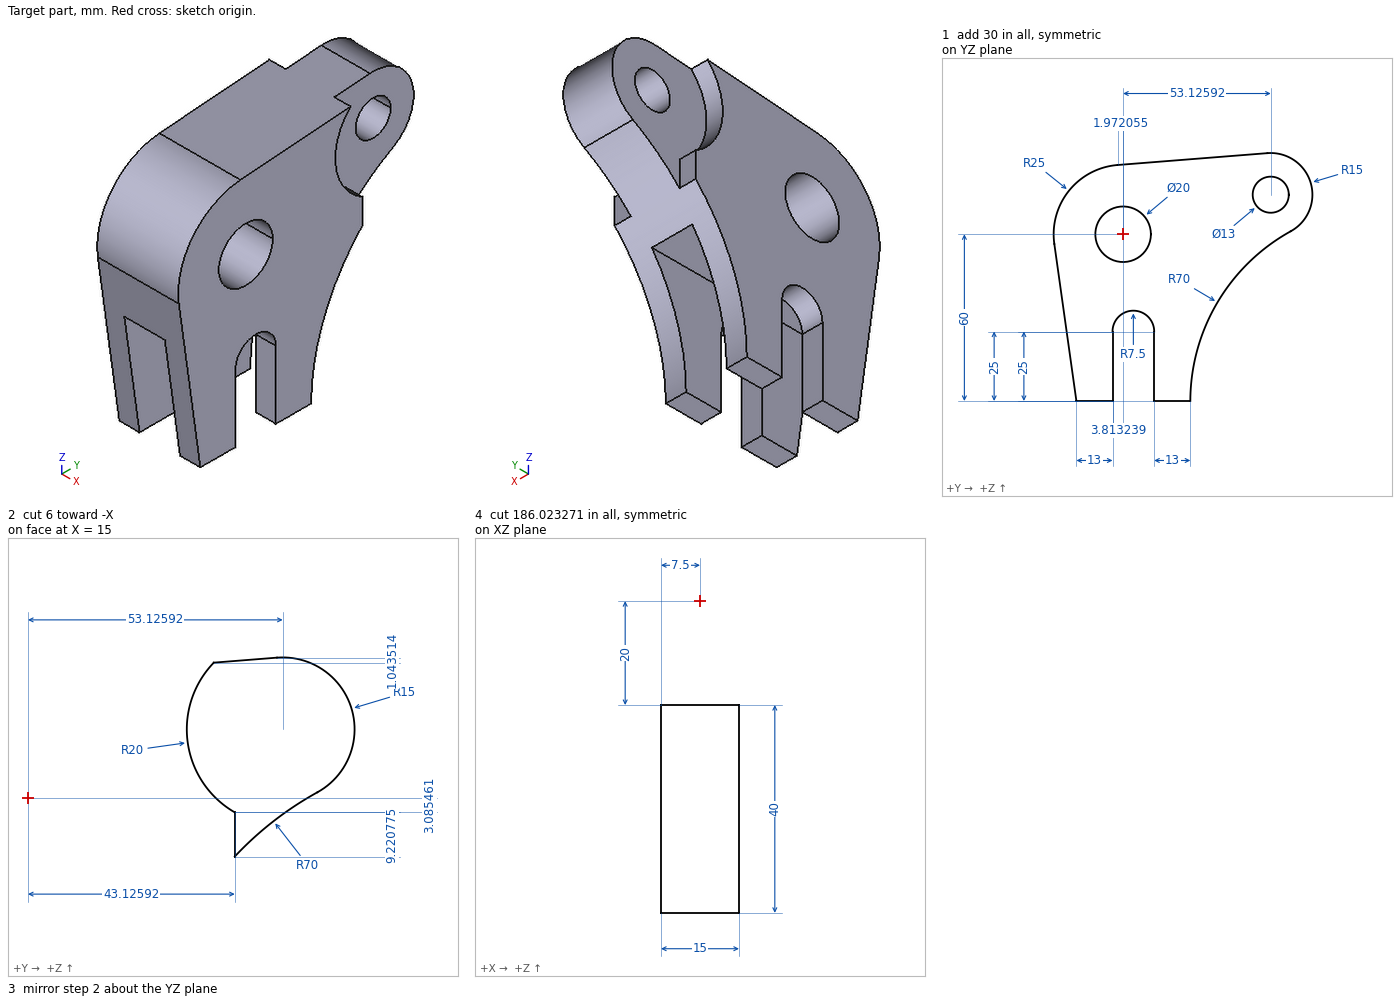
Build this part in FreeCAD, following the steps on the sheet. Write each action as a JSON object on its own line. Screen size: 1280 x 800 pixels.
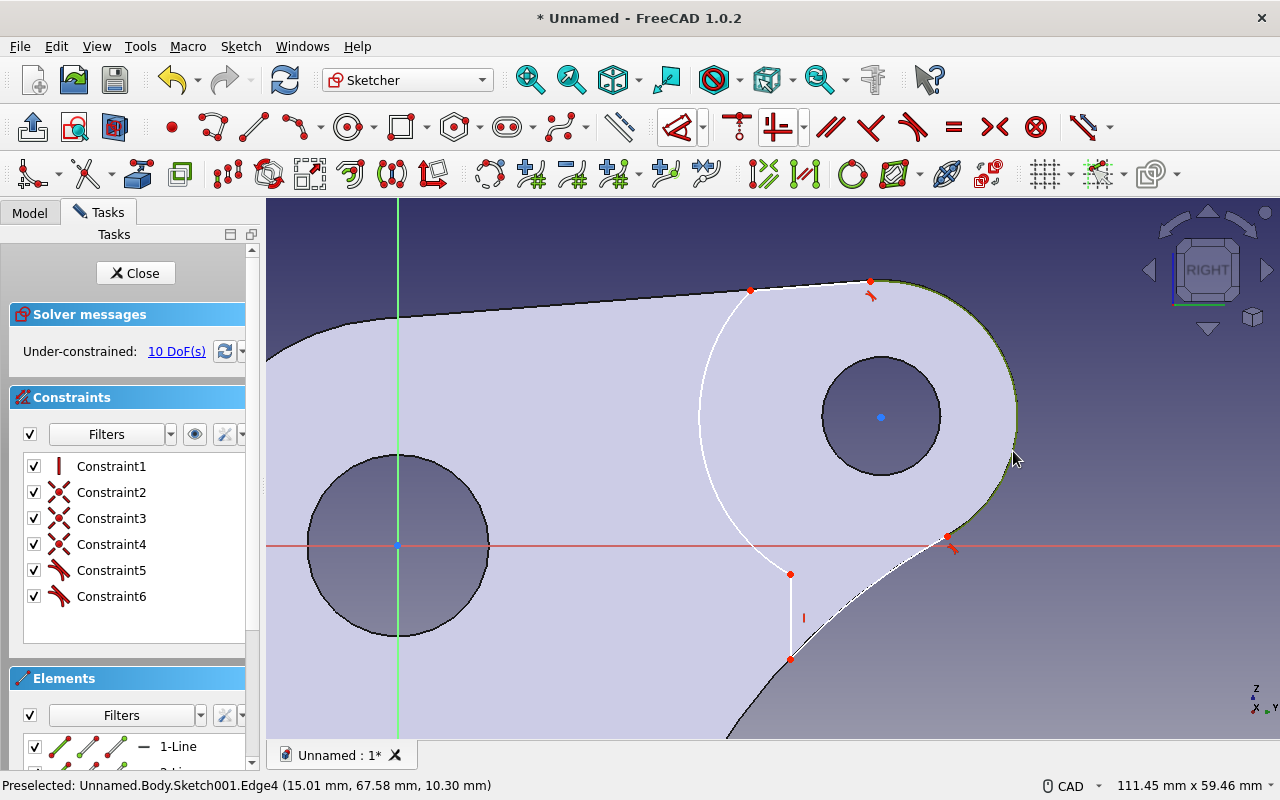
{"action": "left_click", "coordinate": [704, 377]}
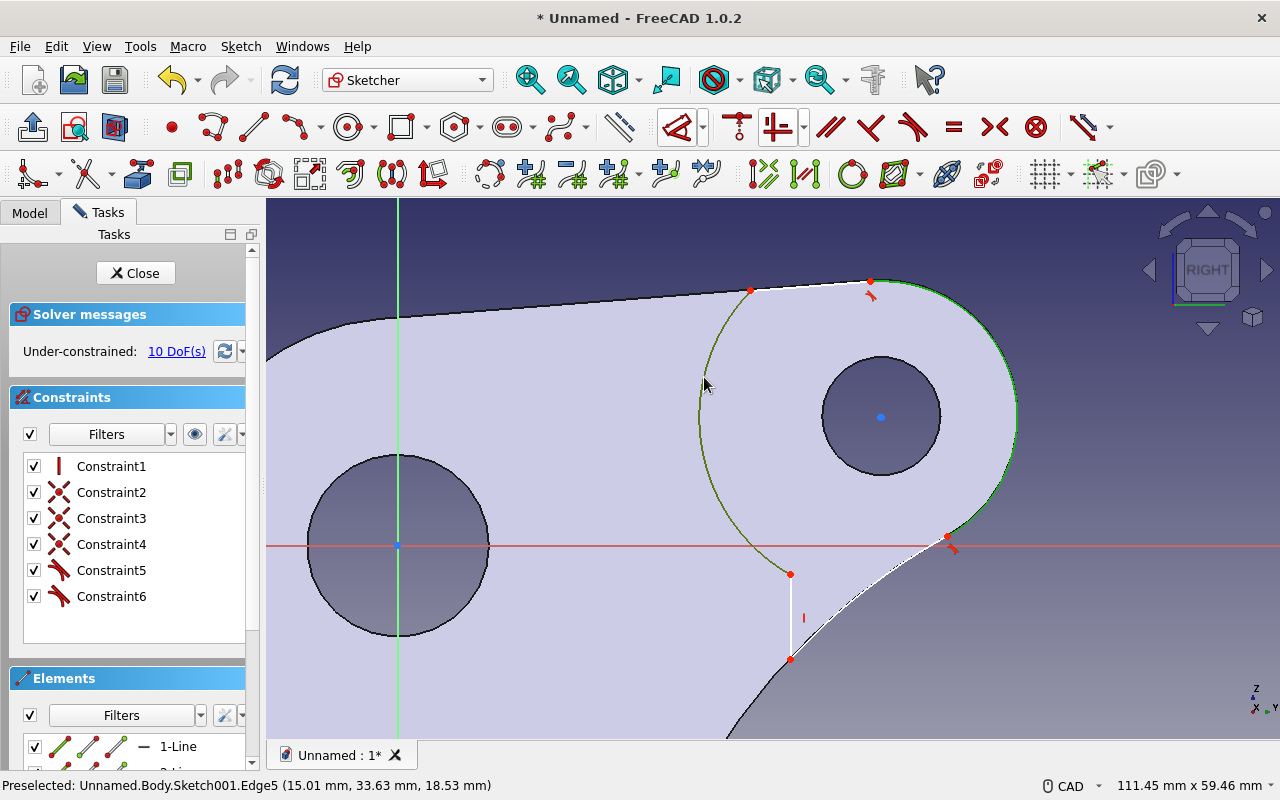
{"action": "left_click", "coordinate": [737, 128]}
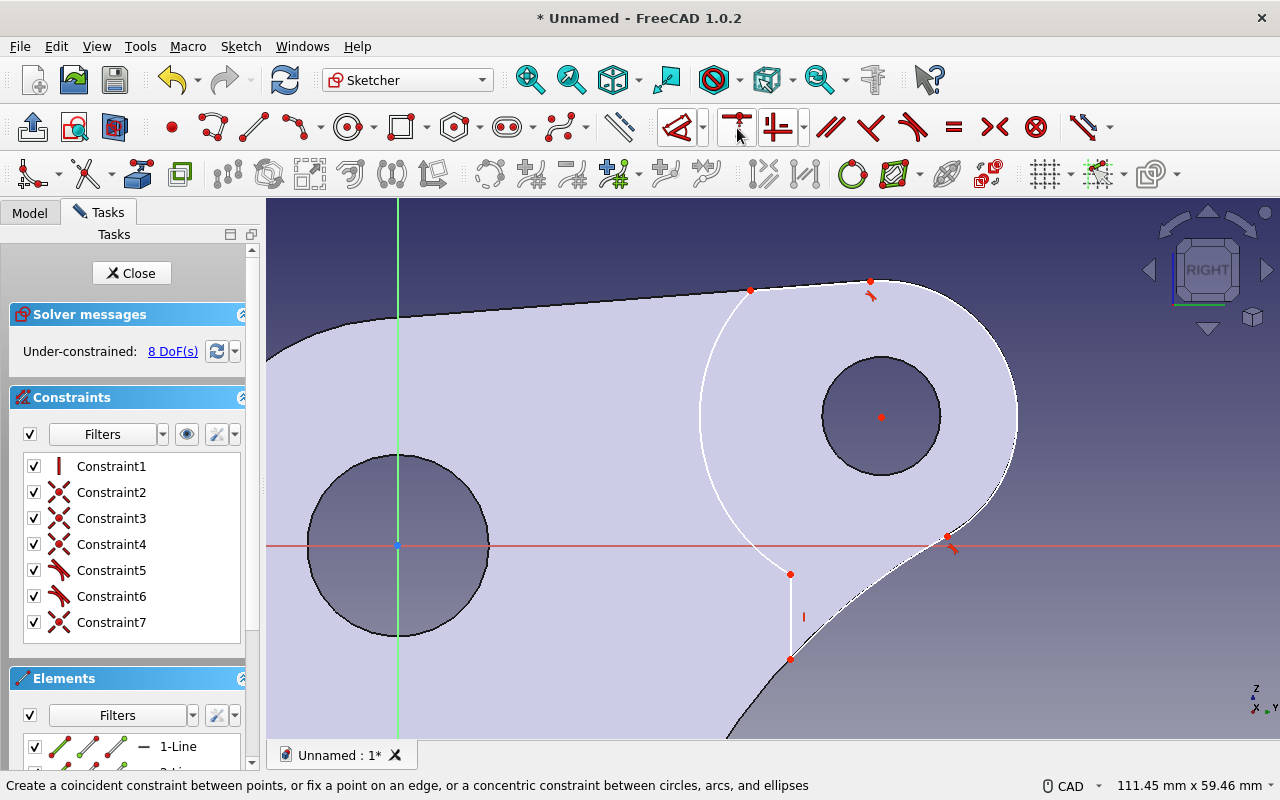
{"action": "left_click", "coordinate": [896, 568]}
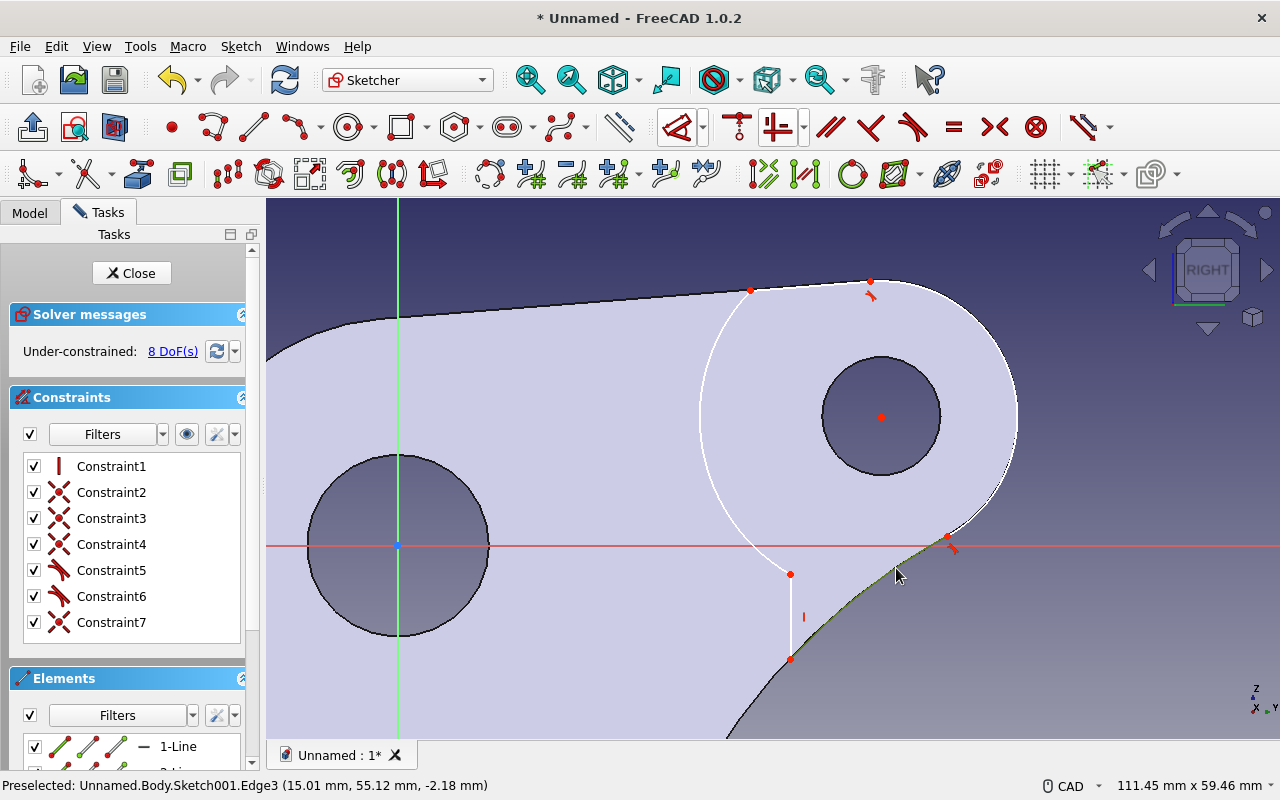
{"action": "left_click", "coordinate": [702, 128]}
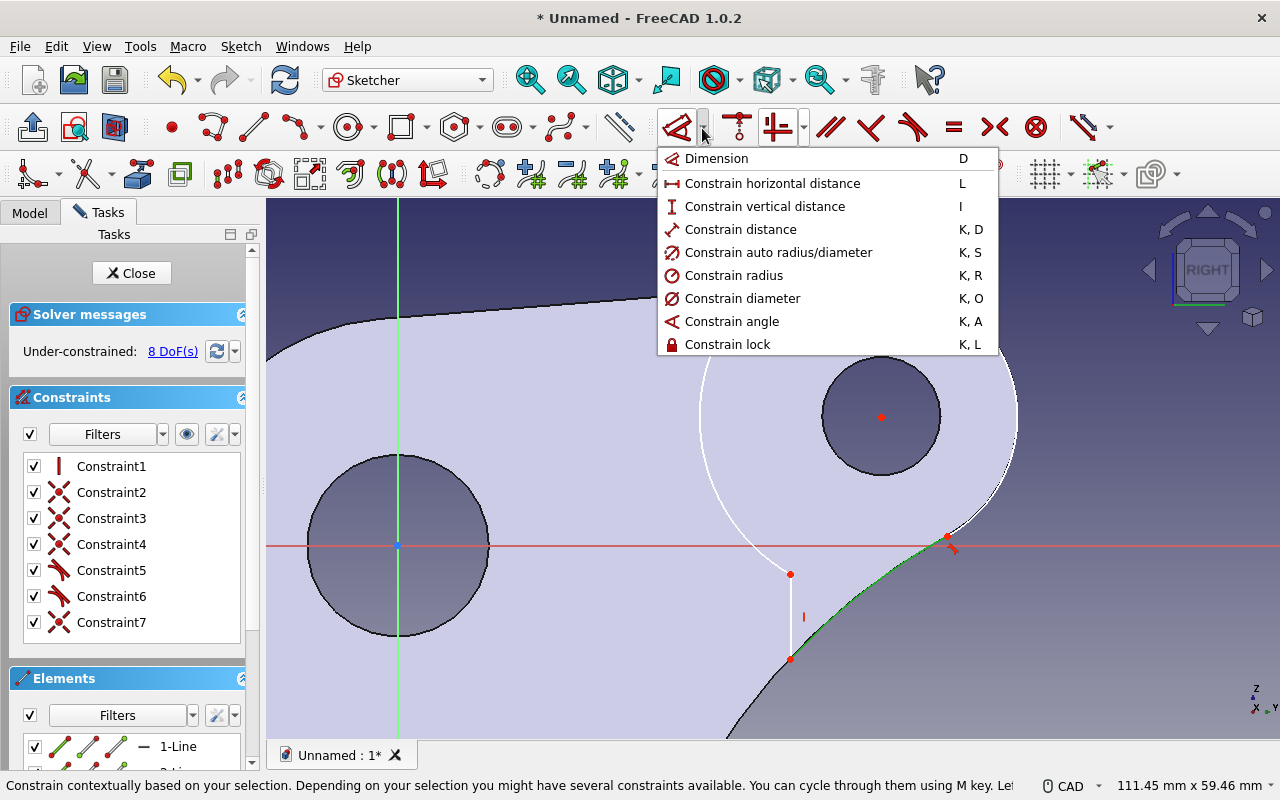
{"action": "left_click", "coordinate": [828, 276]}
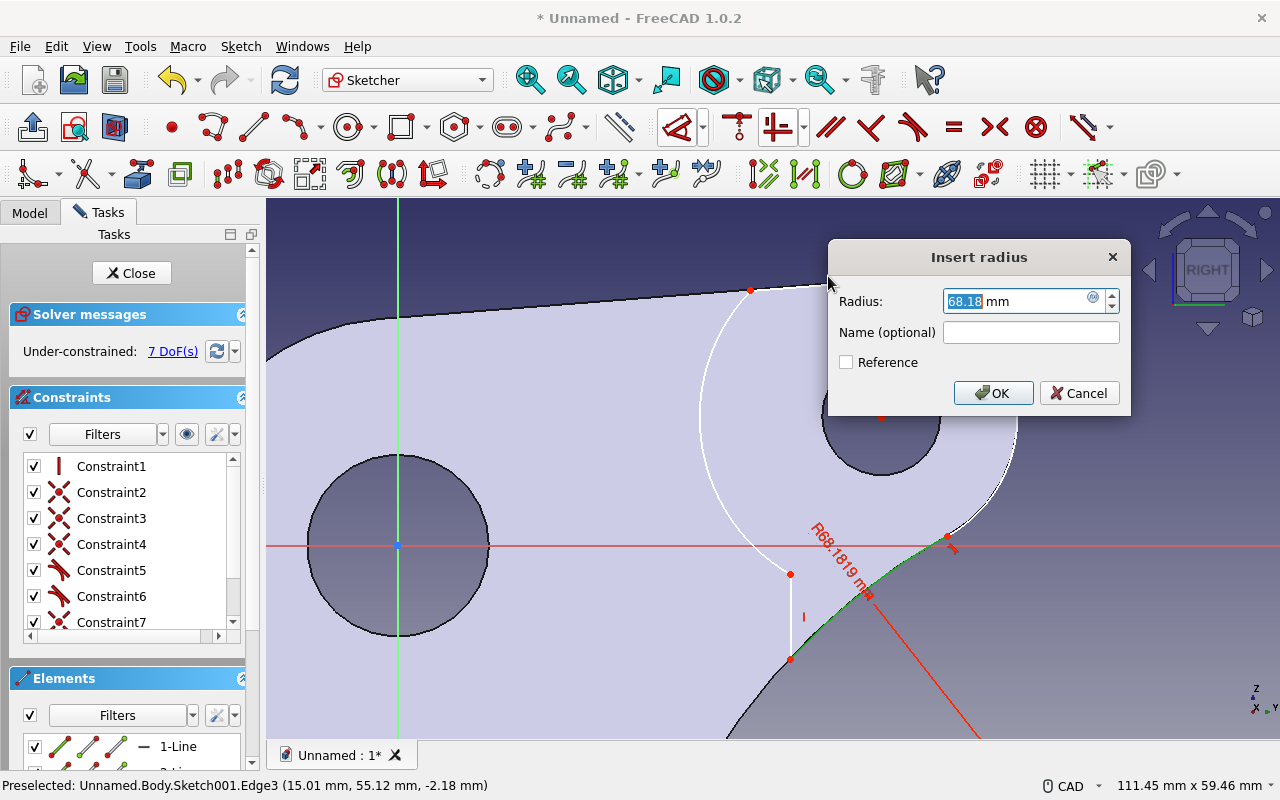
{"action": "type", "text": "70"}
{"action": "key", "text": "Return"}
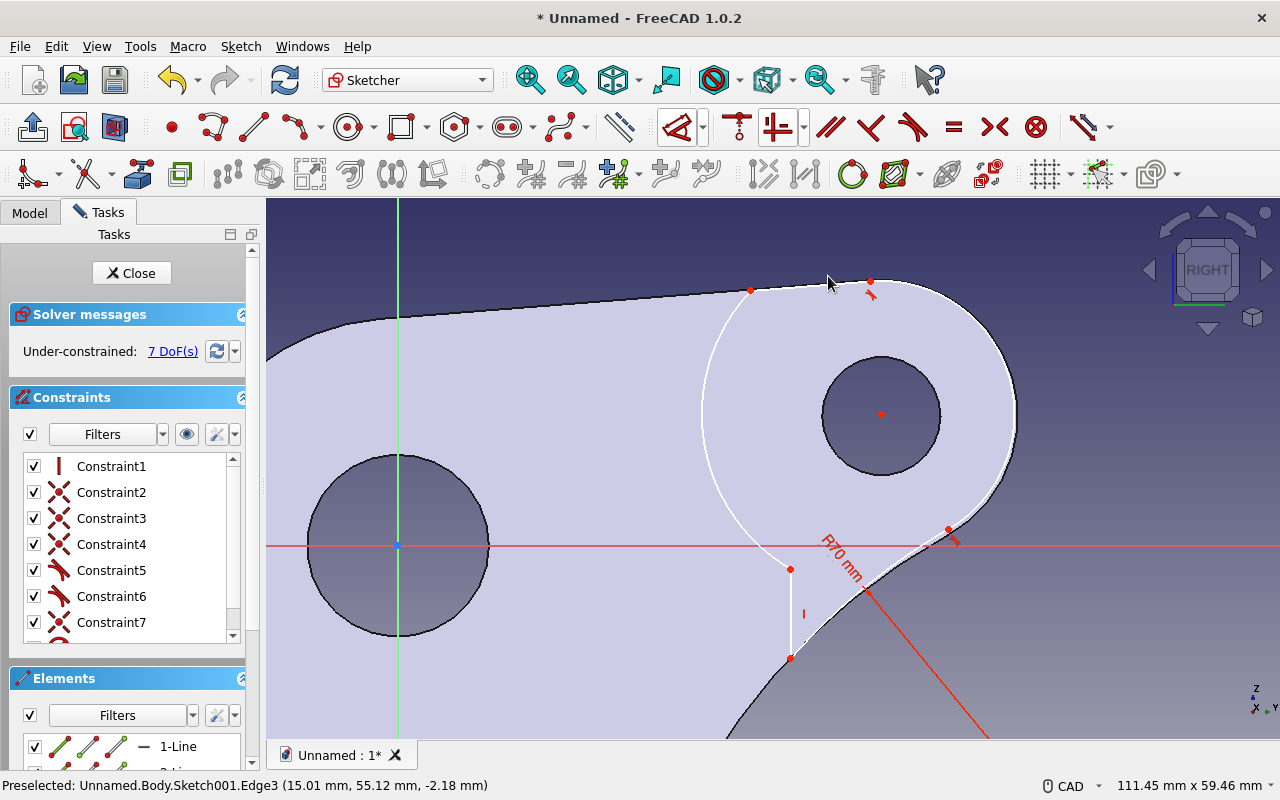
{"action": "left_click", "coordinate": [1011, 445]}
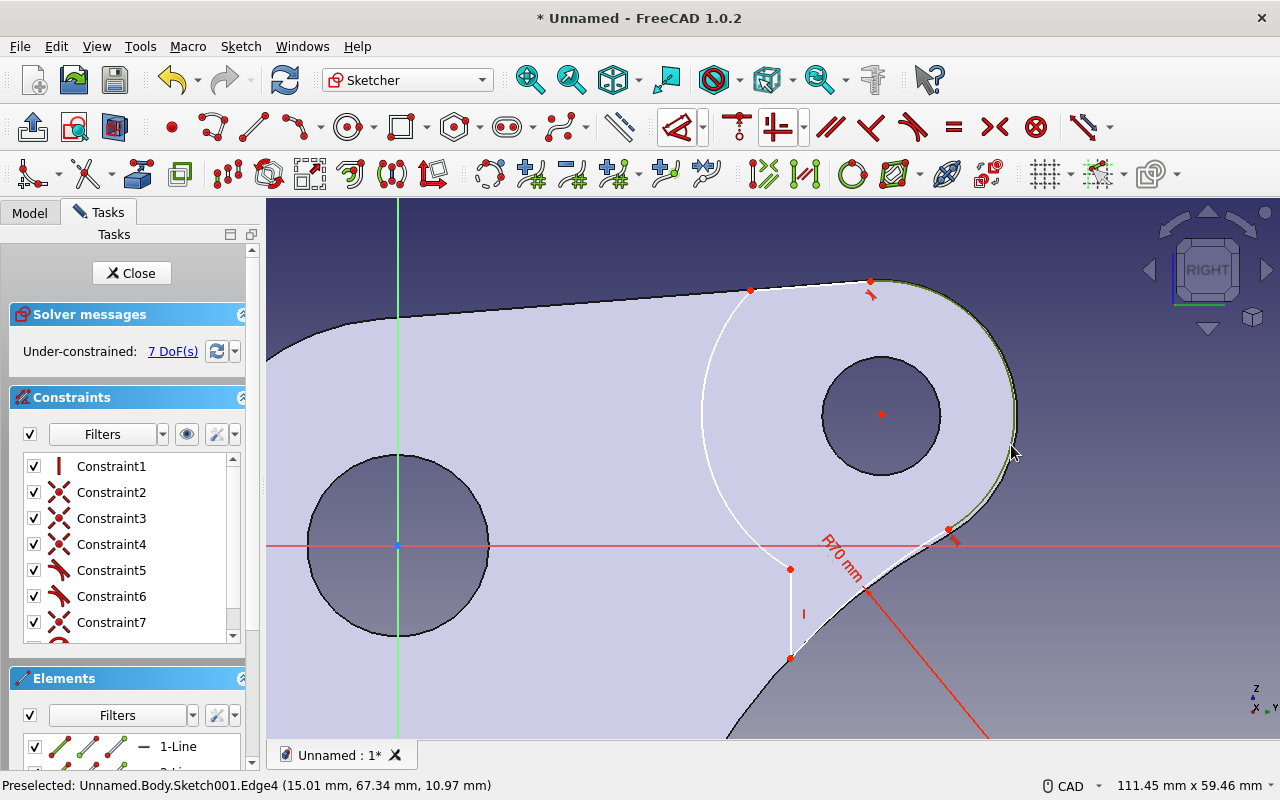
{"action": "key", "text": "k r"}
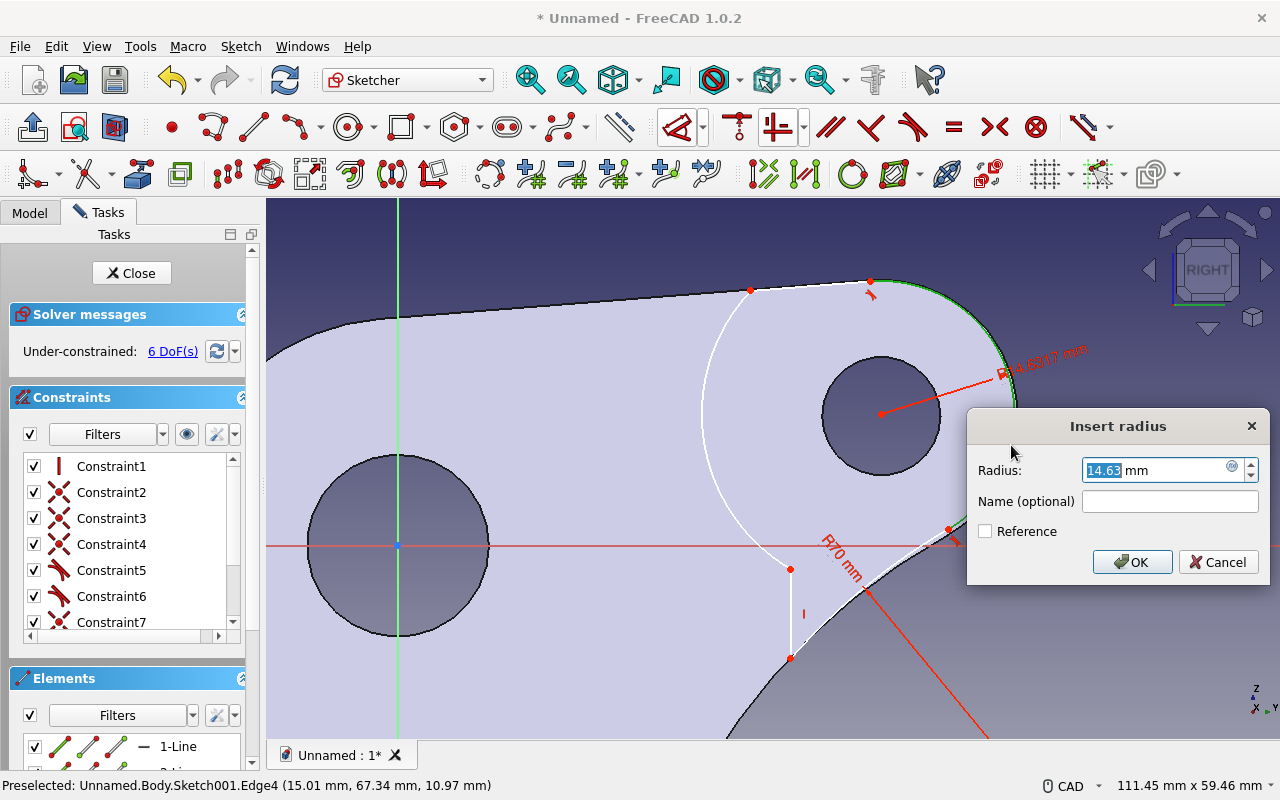
{"action": "type", "text": "15"}
{"action": "key", "text": "Return"}